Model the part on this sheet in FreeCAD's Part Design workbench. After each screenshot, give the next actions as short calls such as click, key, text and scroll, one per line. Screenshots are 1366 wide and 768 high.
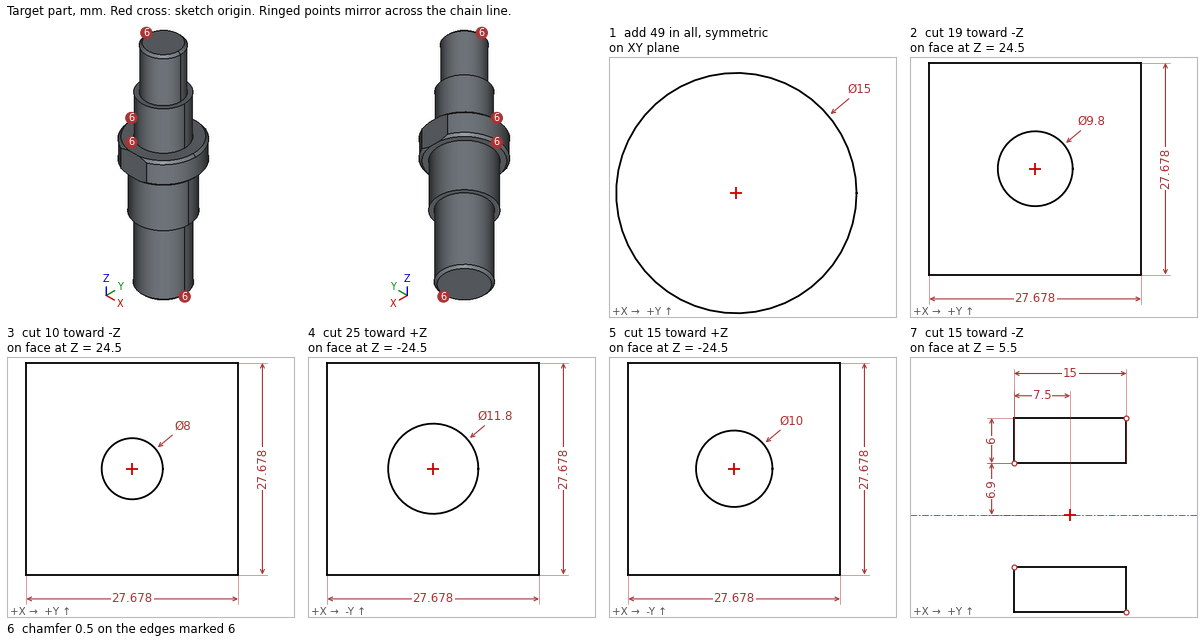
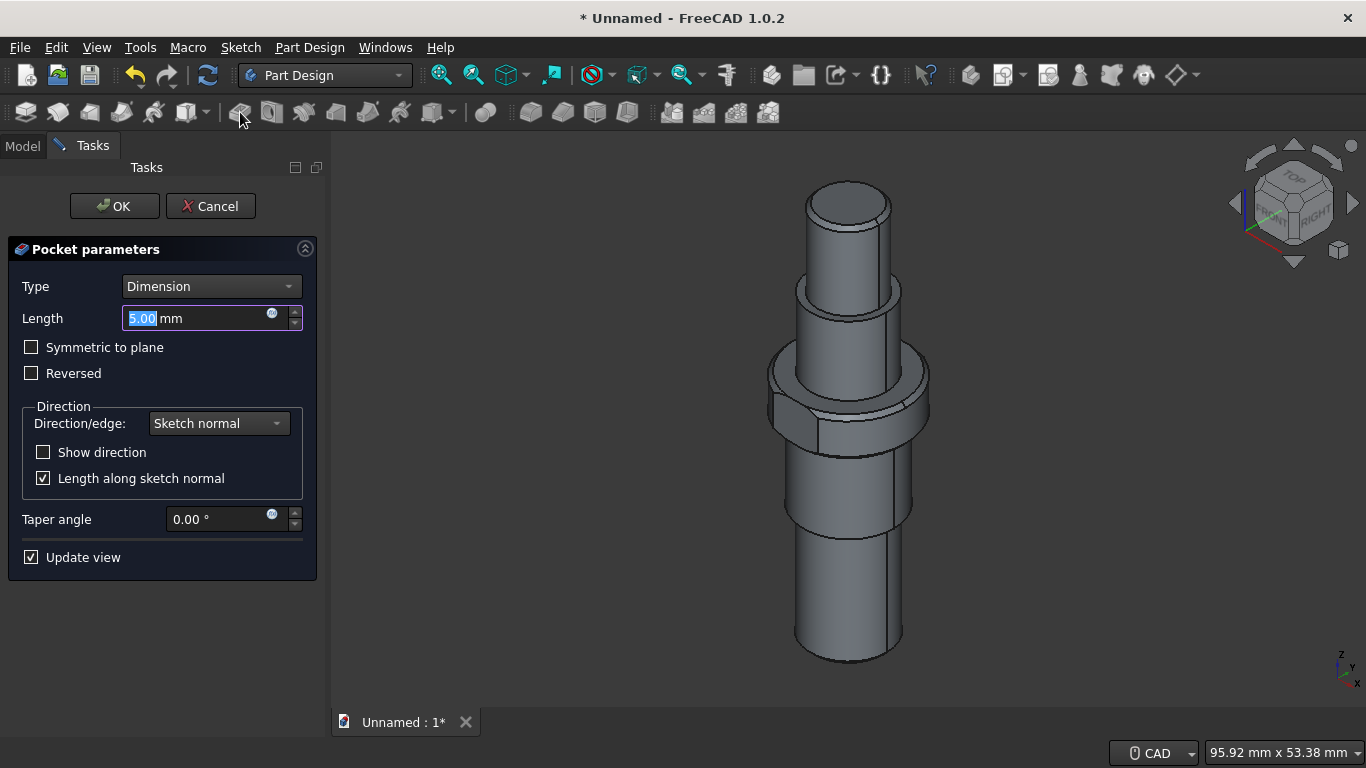
text(15)
key(Tab)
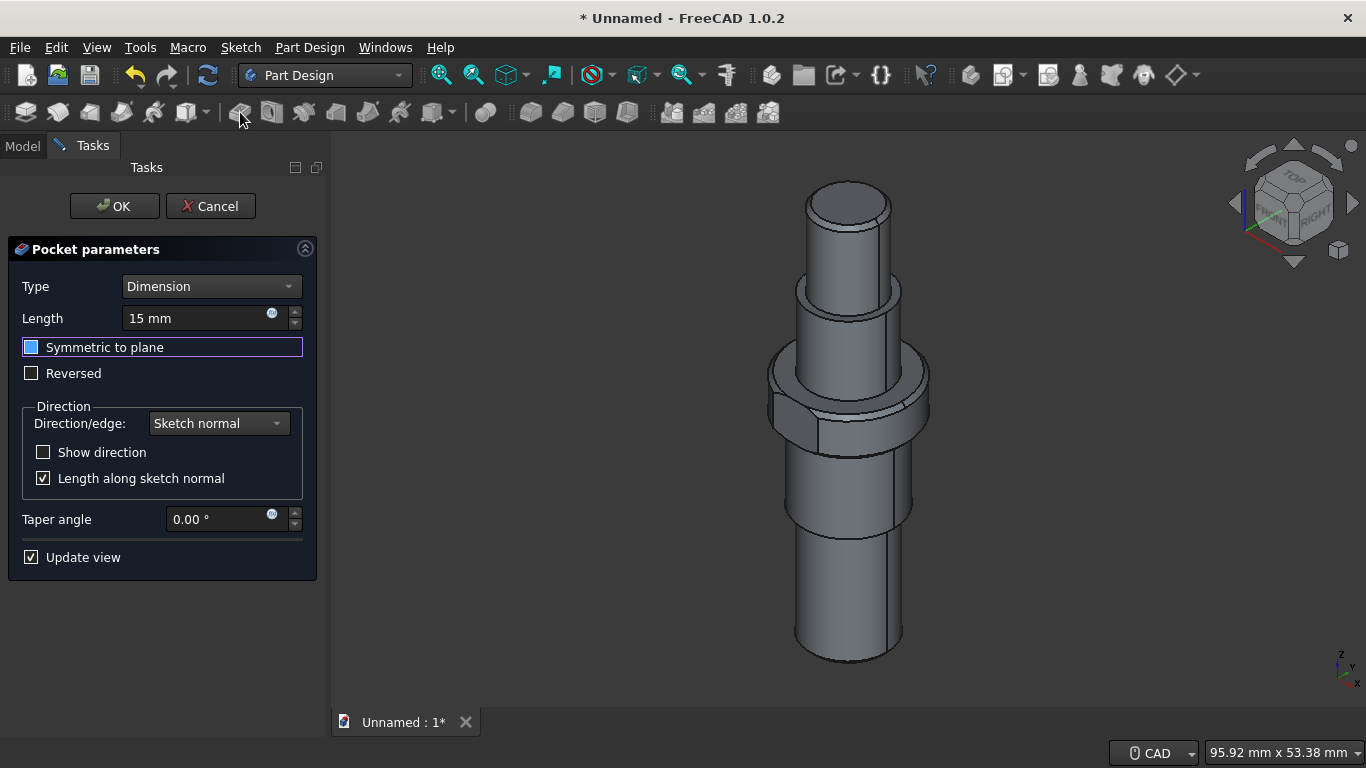
click(115, 206)